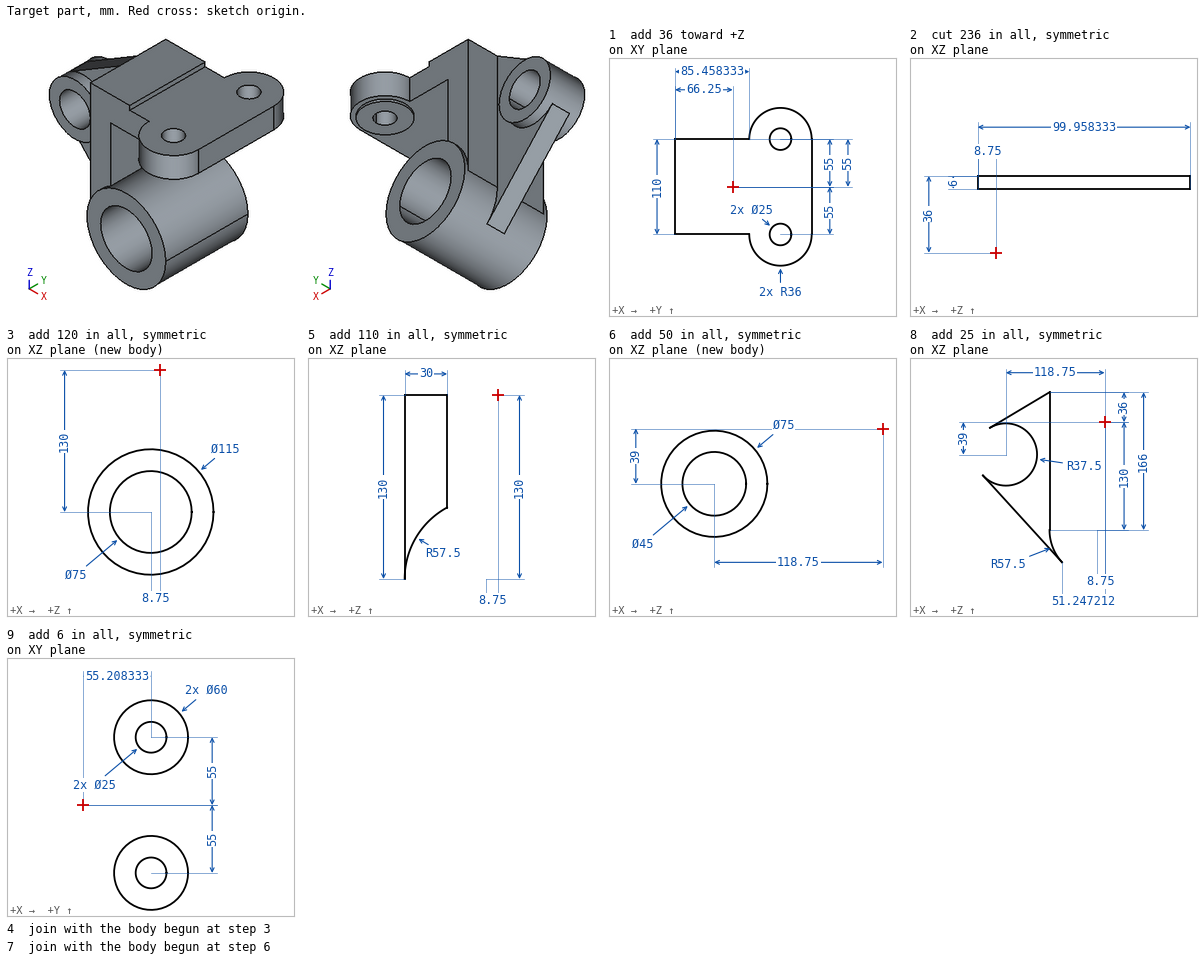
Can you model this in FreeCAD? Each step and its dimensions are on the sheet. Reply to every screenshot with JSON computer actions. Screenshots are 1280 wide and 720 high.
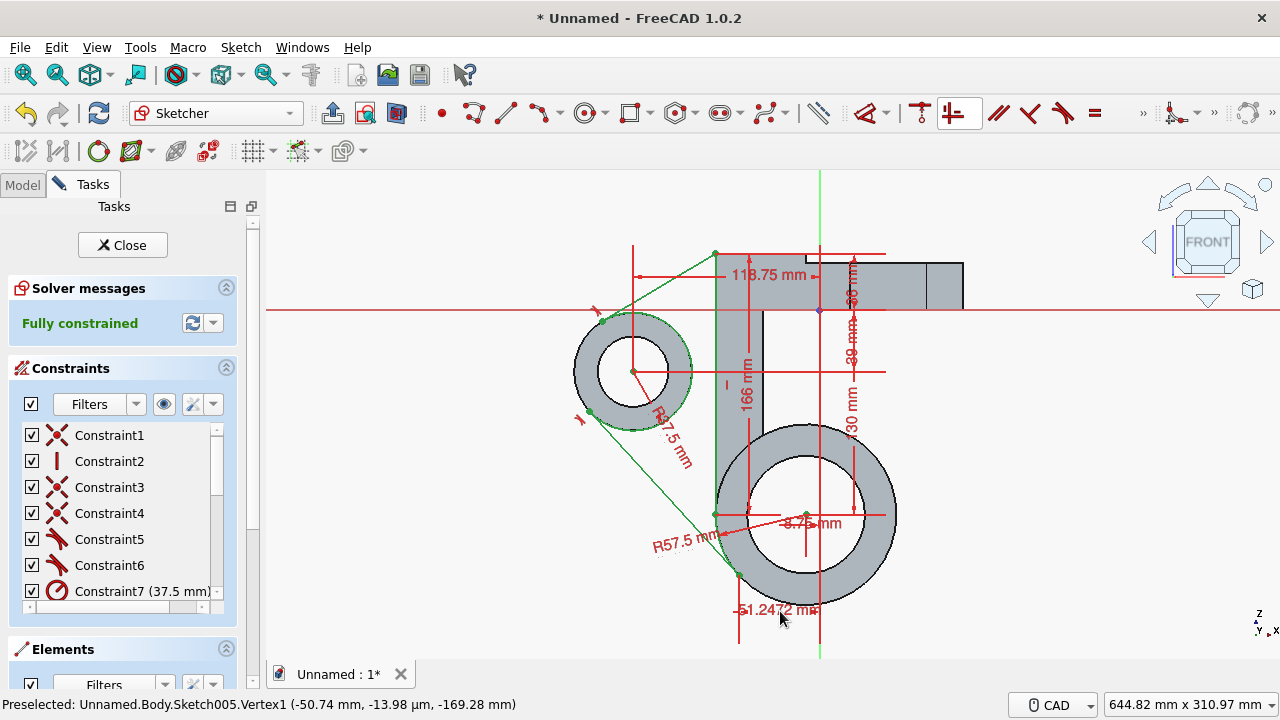
{"action": "left_click", "coordinate": [123, 245]}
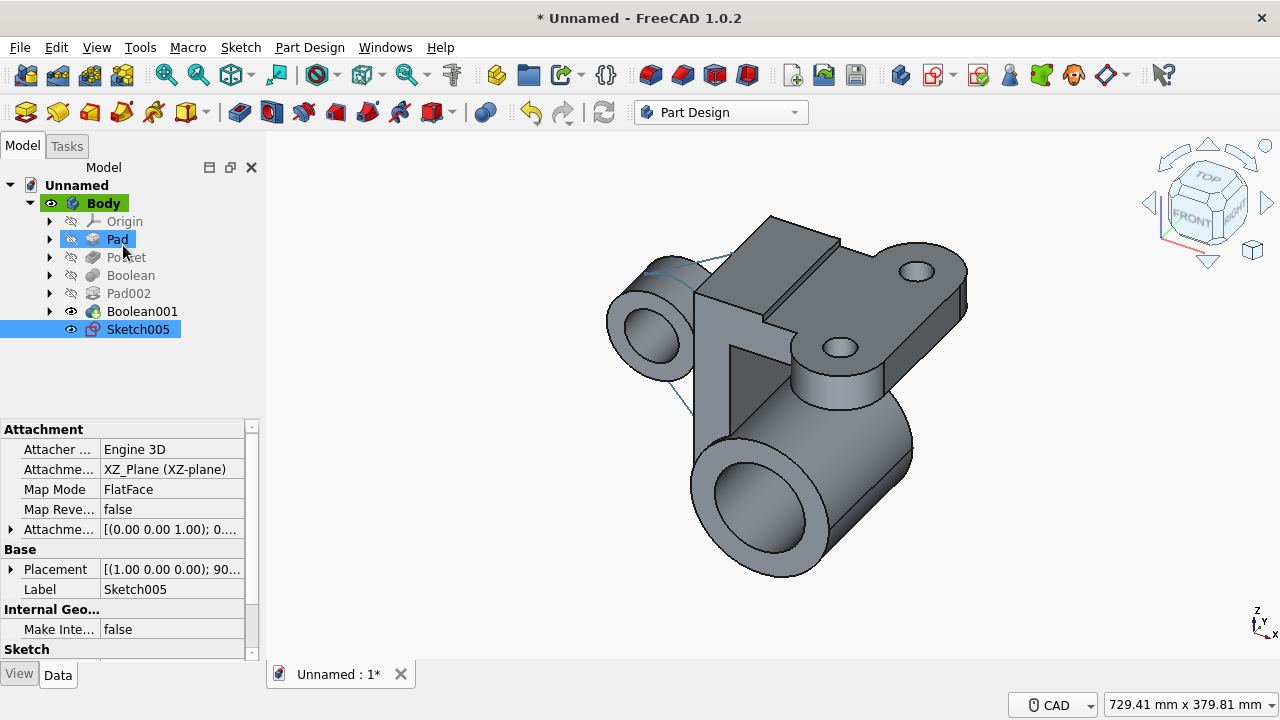
{"action": "left_click", "coordinate": [26, 112]}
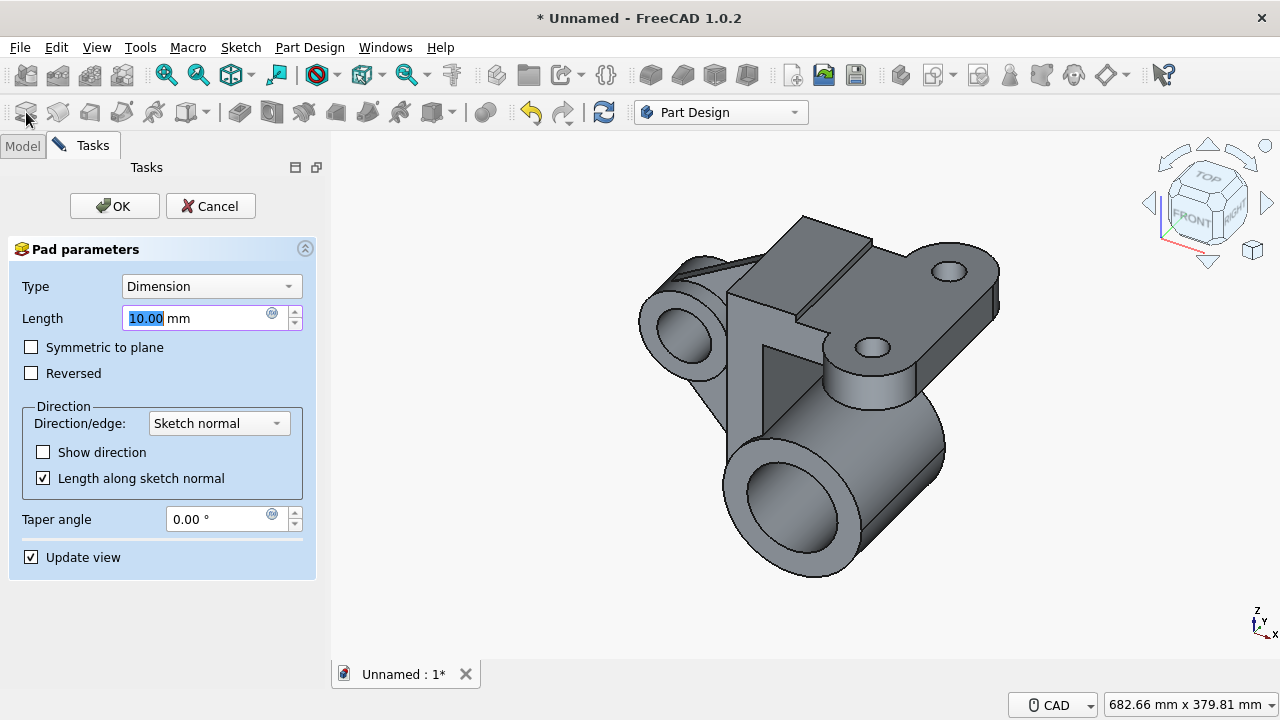
{"action": "type", "text": "25"}
{"action": "key", "text": "Tab"}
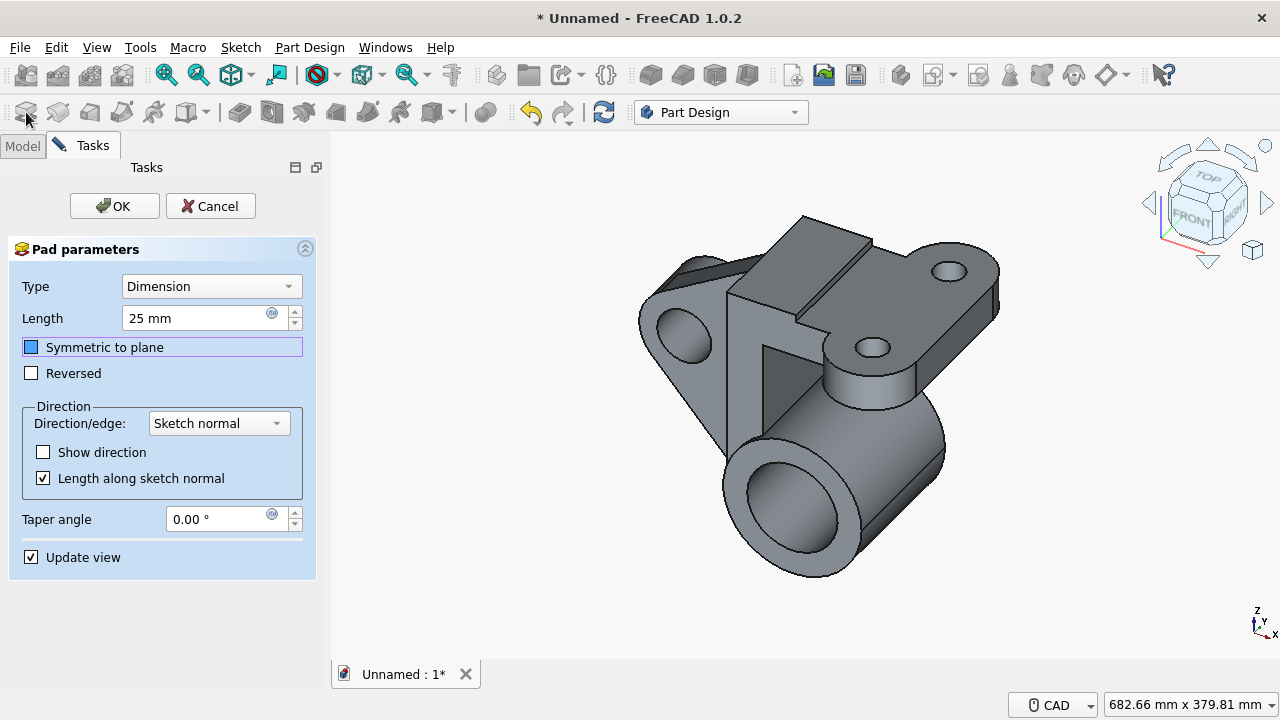
{"action": "left_click", "coordinate": [30, 347]}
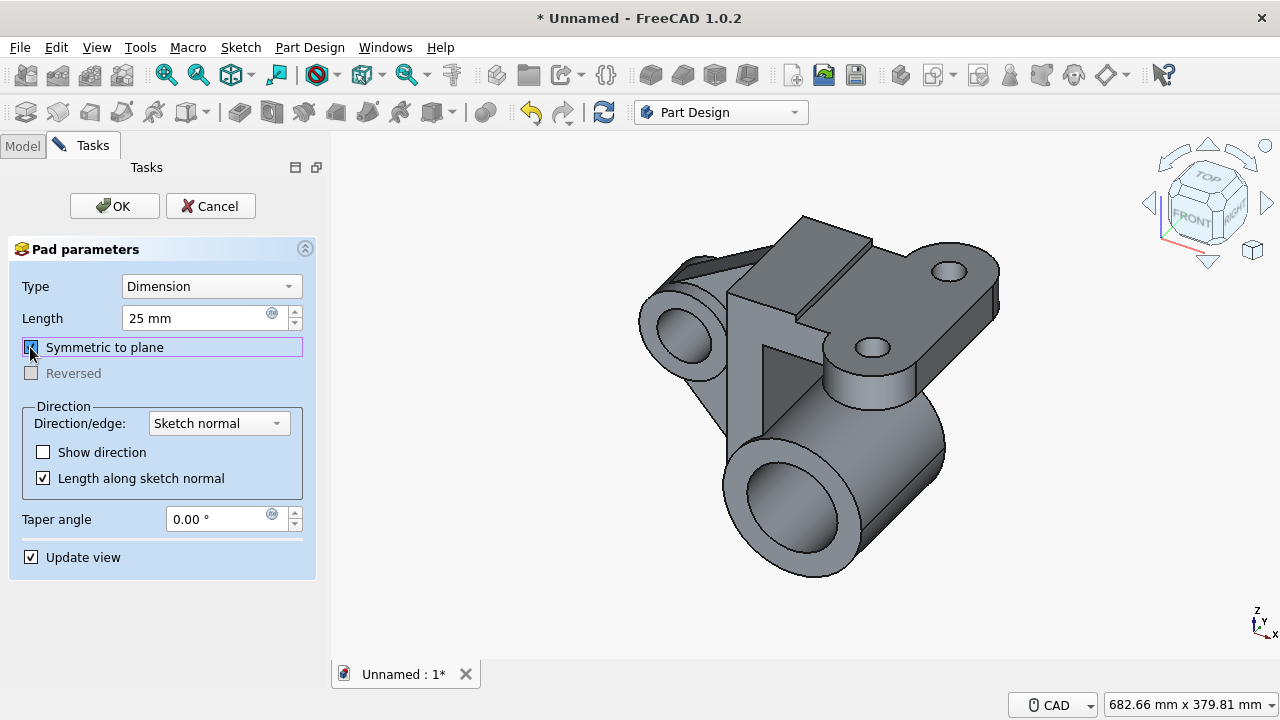
{"action": "left_click", "coordinate": [115, 206]}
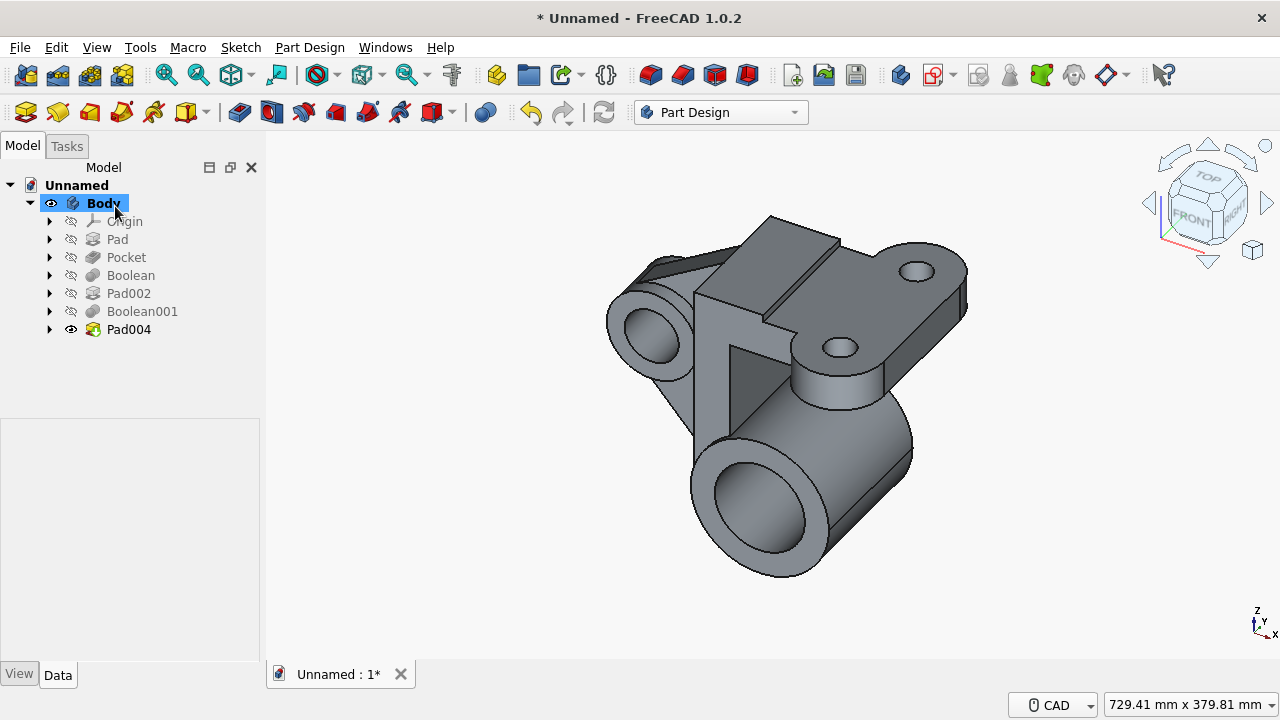
{"action": "left_click", "coordinate": [934, 76]}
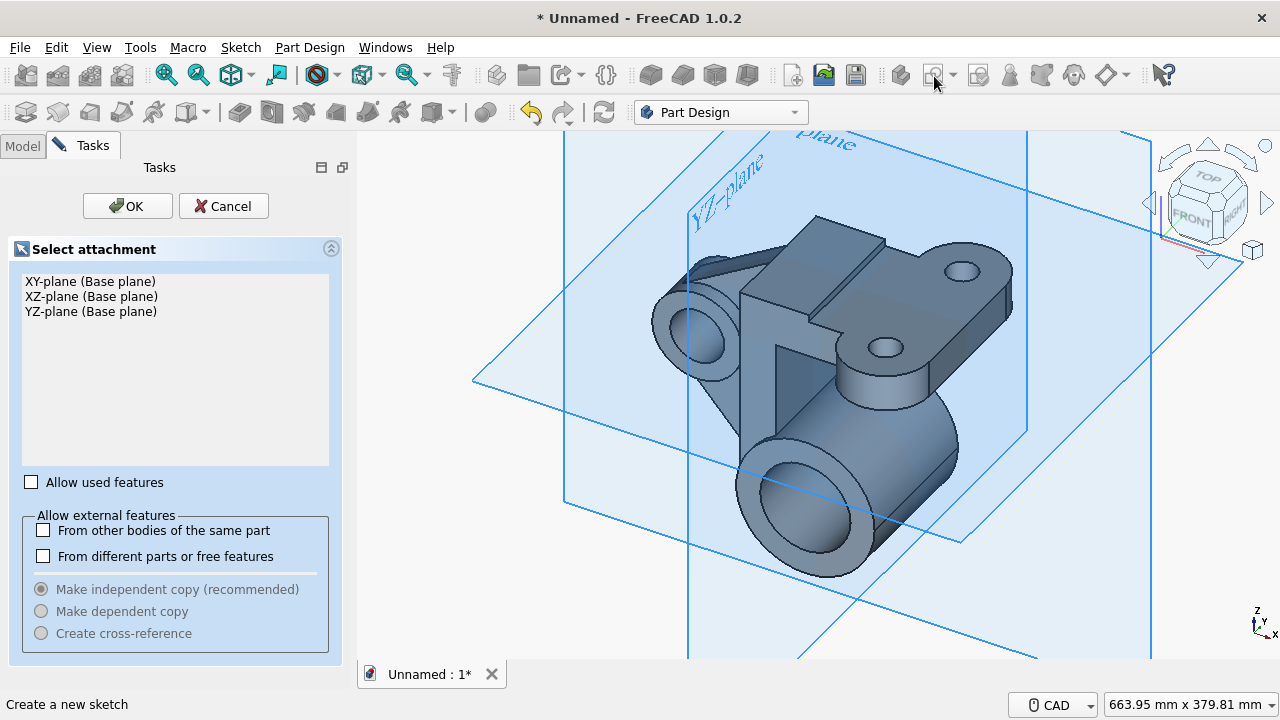
{"action": "left_click", "coordinate": [82, 282]}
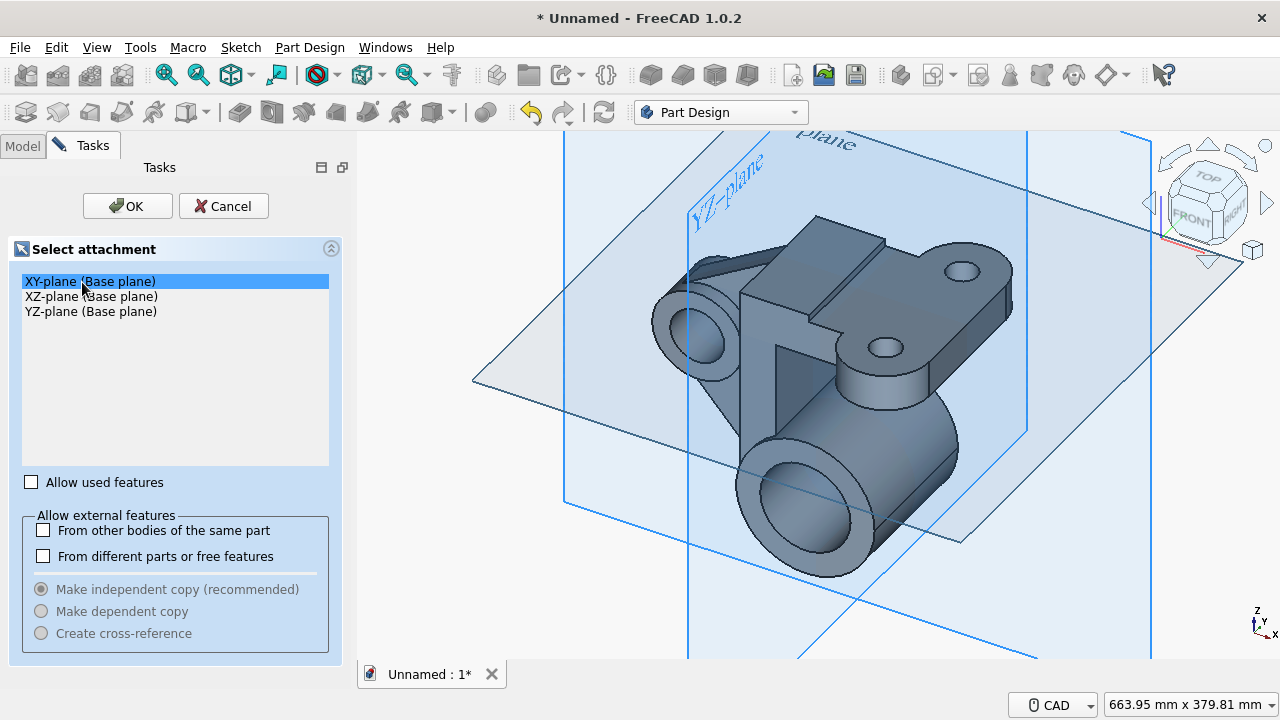
{"action": "left_click", "coordinate": [128, 206]}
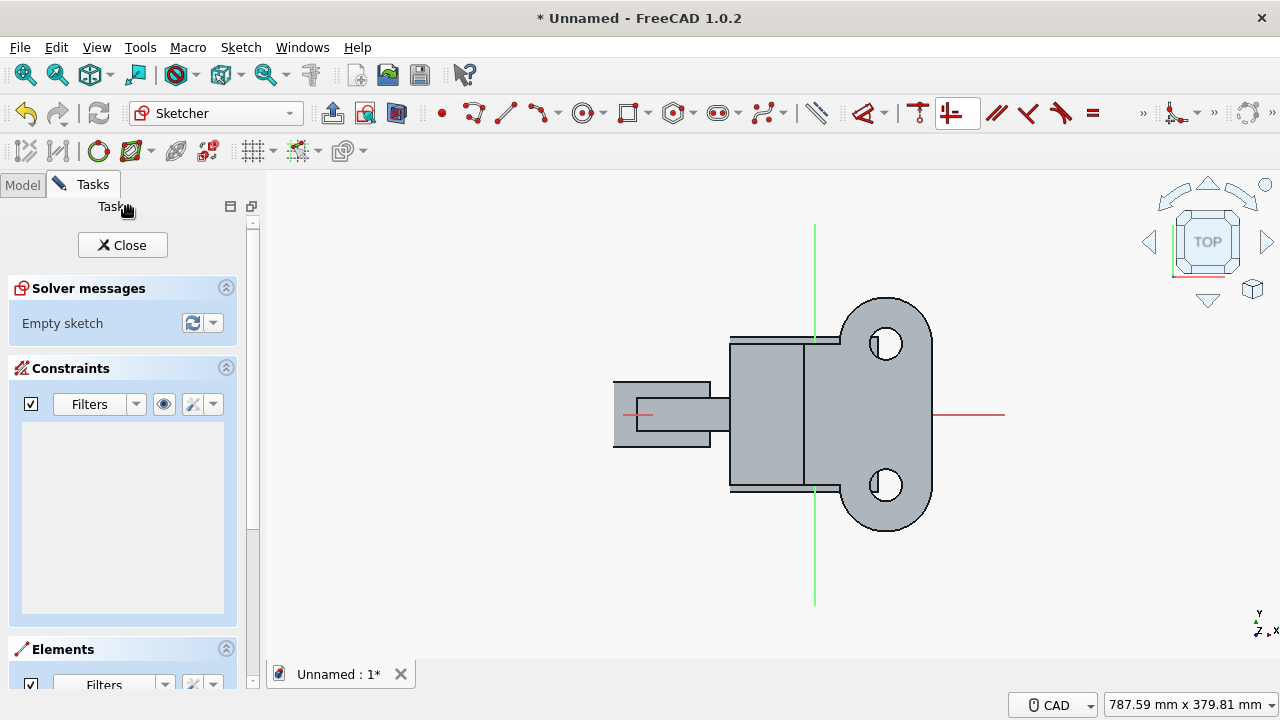
{"action": "left_click", "coordinate": [398, 114]}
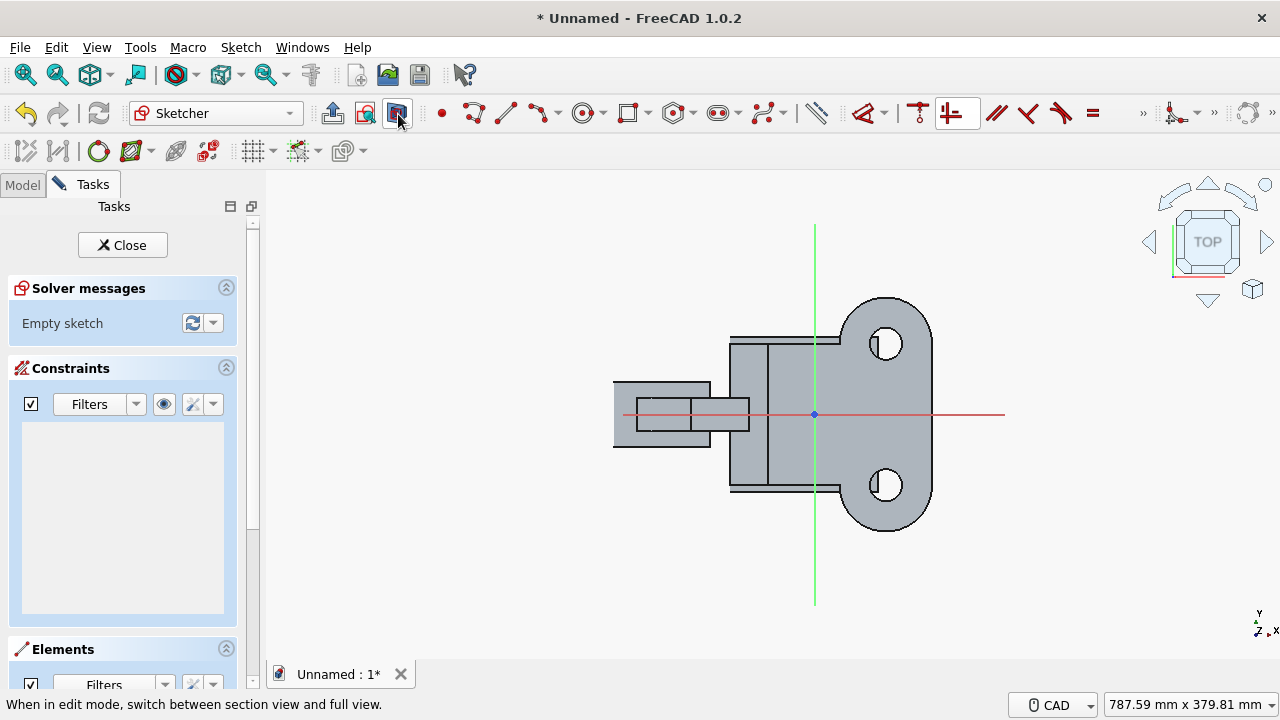
{"action": "scroll", "coordinate": [1115, 414], "scroll_direction": "up", "scroll_amount": 2}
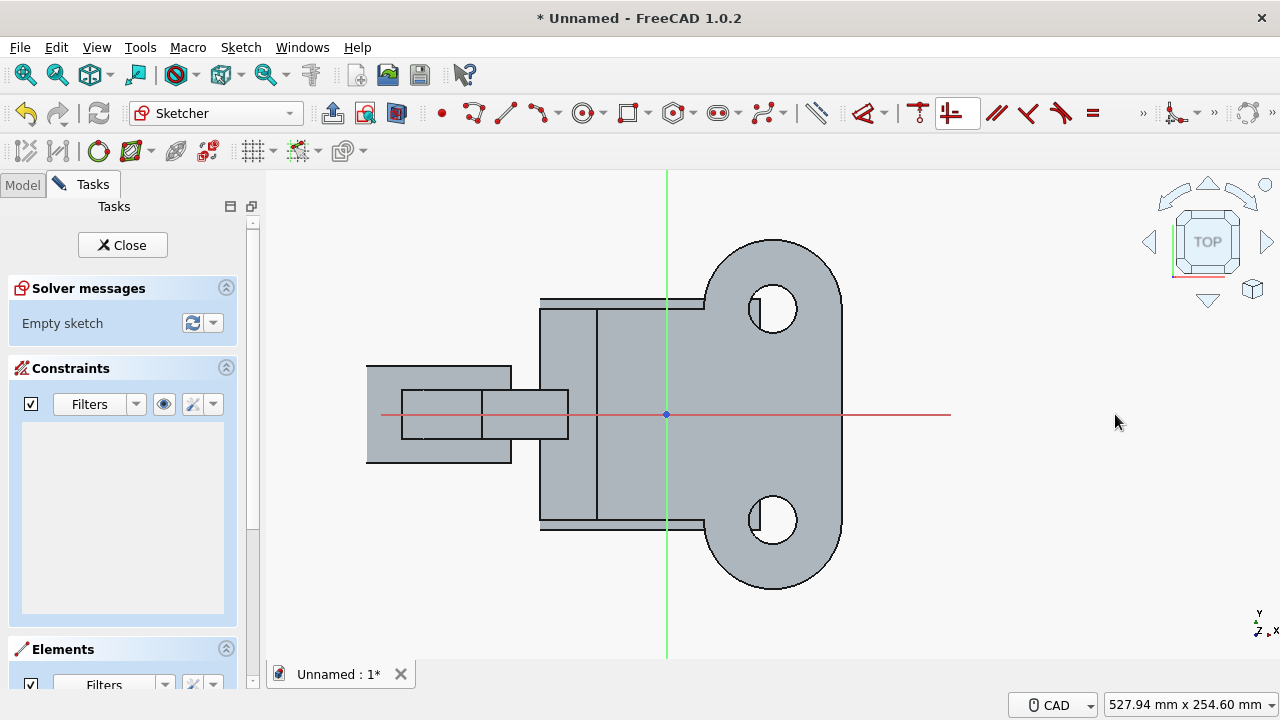
{"action": "left_click", "coordinate": [584, 114]}